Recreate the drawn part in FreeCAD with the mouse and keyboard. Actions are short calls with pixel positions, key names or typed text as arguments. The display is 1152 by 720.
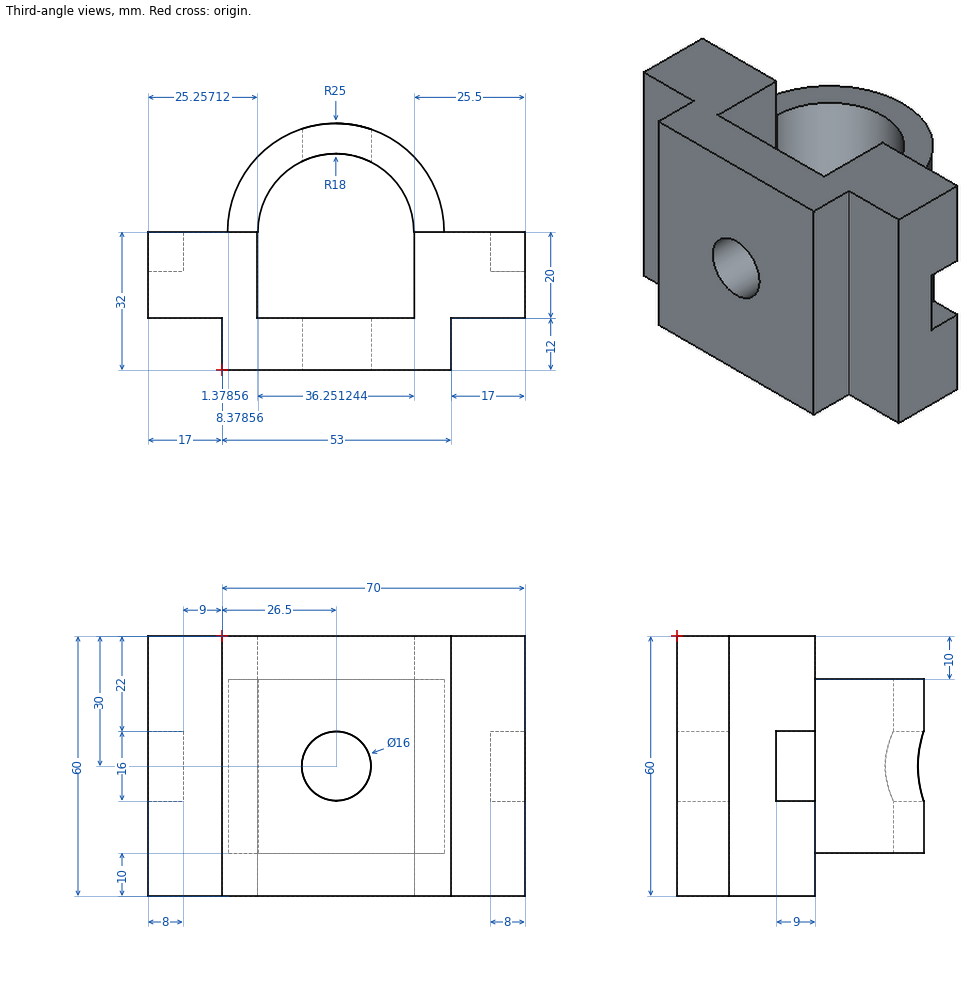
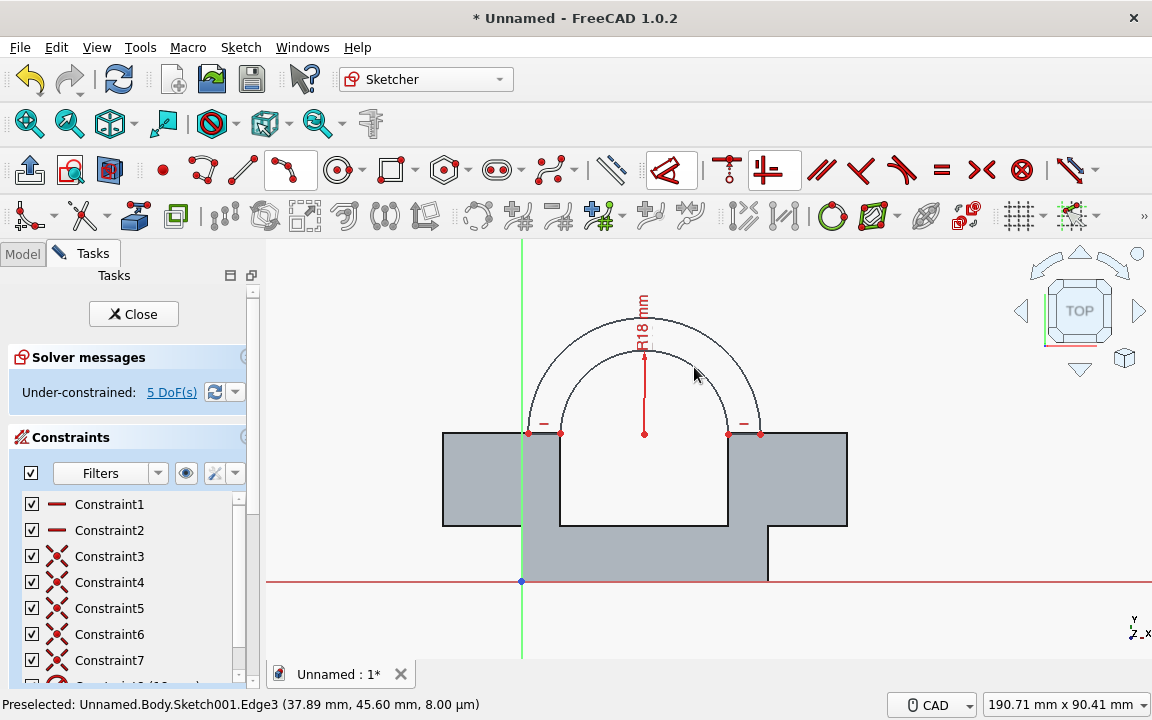
click(713, 340)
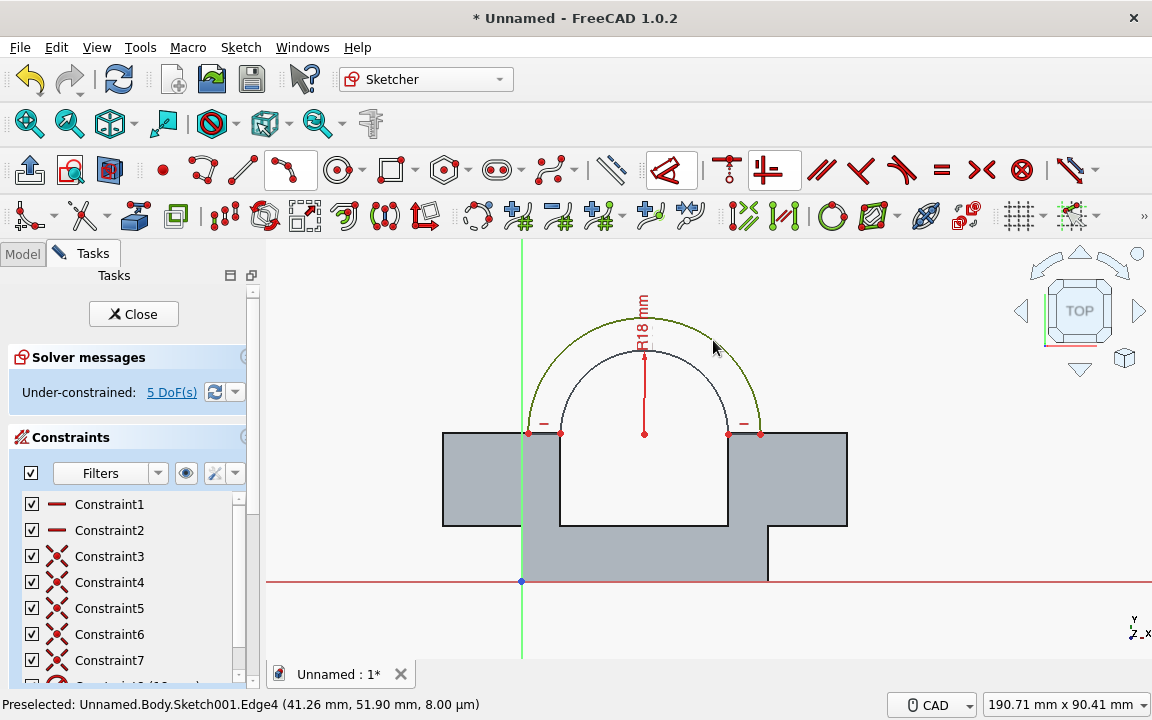
key(k)
key(r)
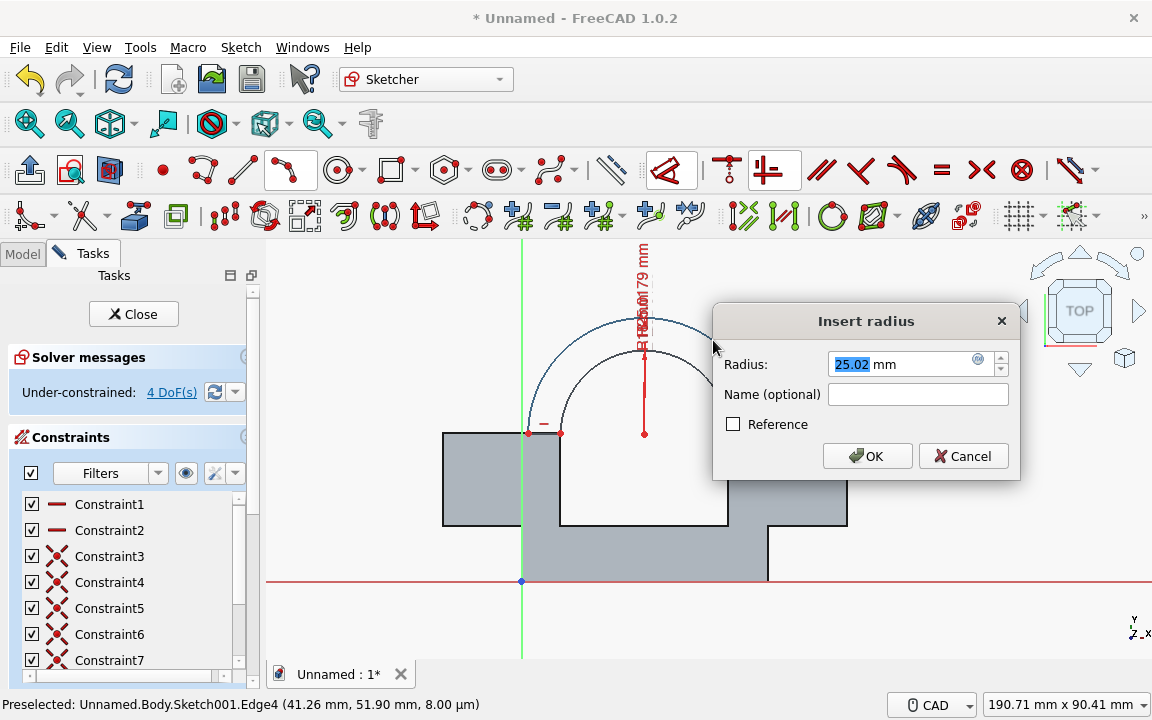
text(25)
key(Return)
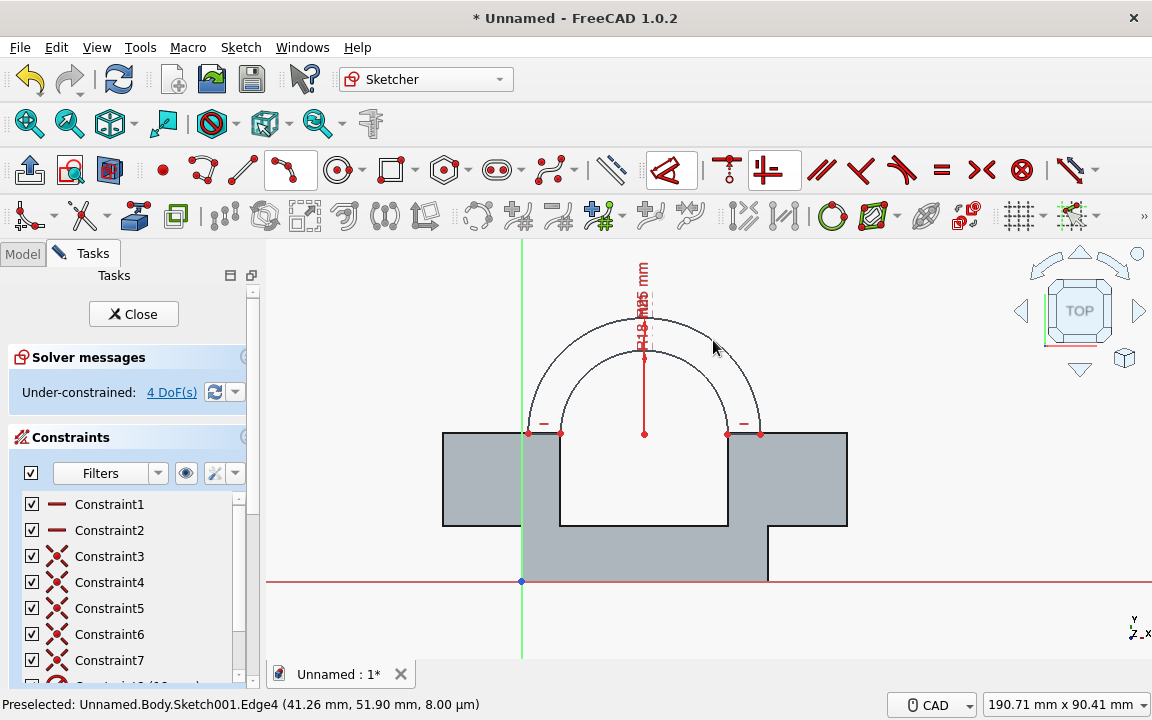
click(528, 434)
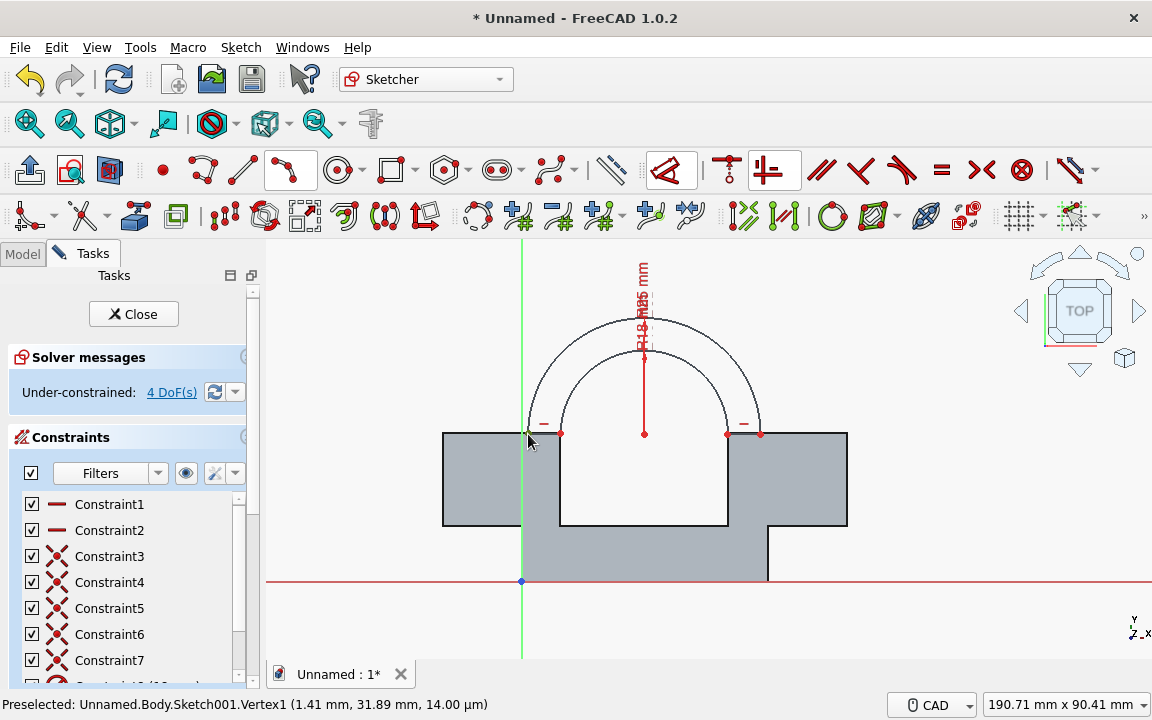
key(i)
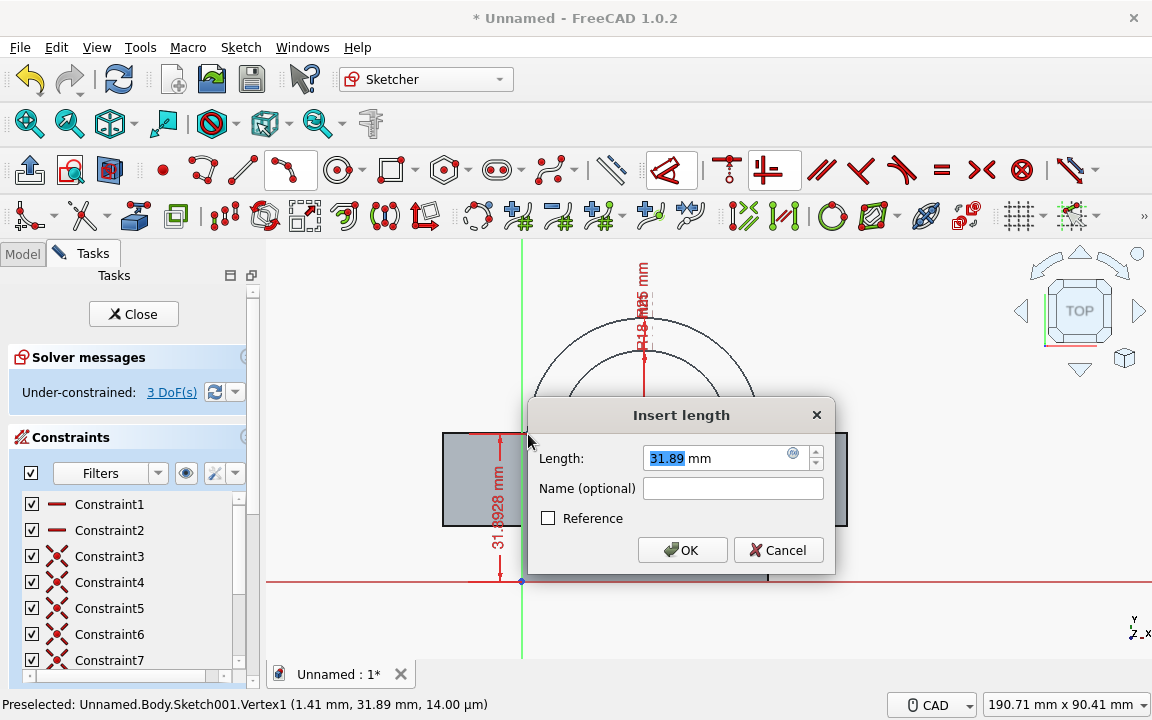
text(32)
key(Return)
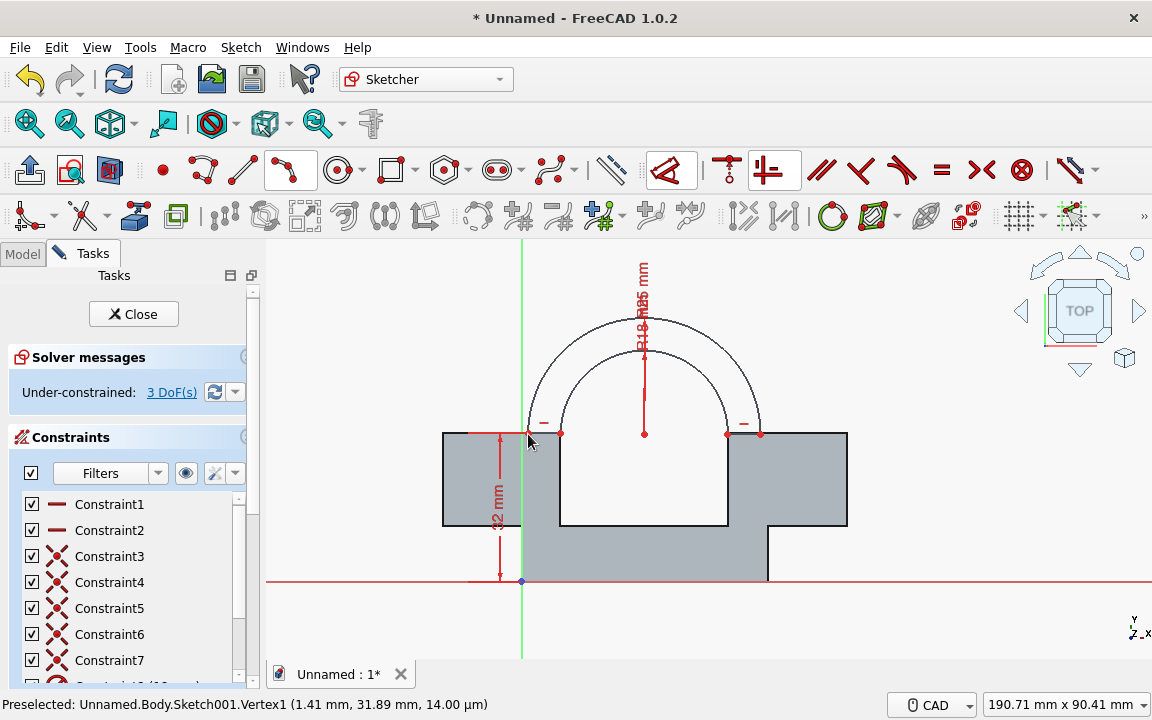
click(728, 434)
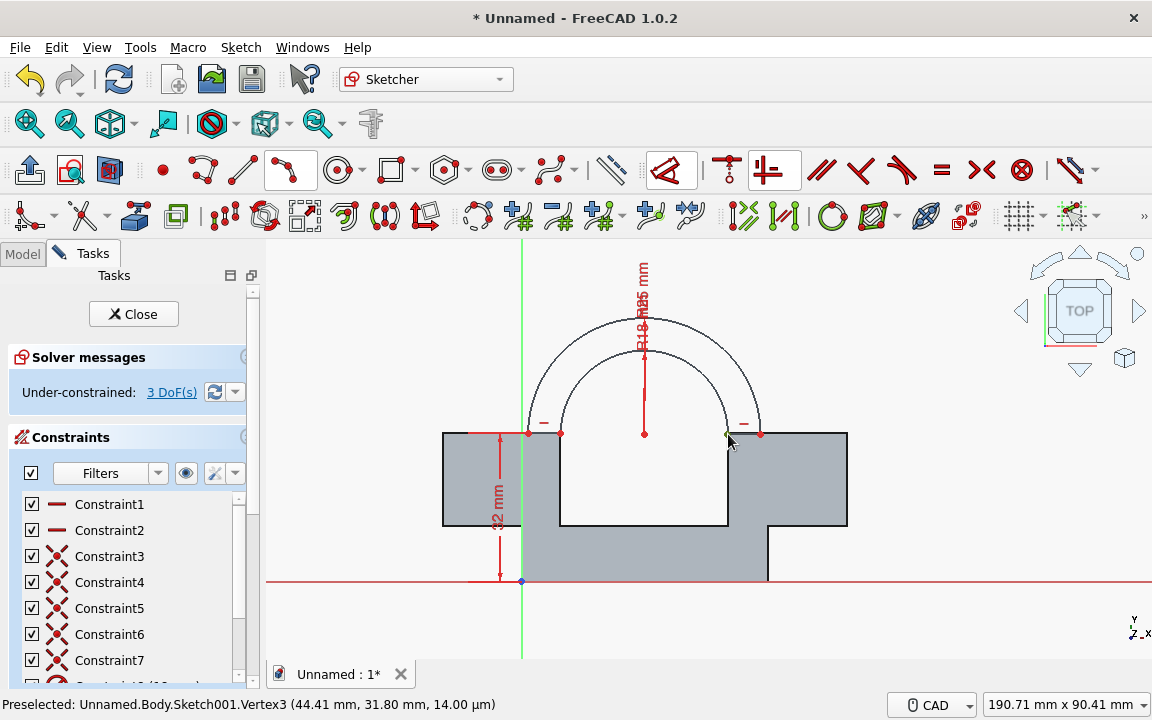
click(692, 170)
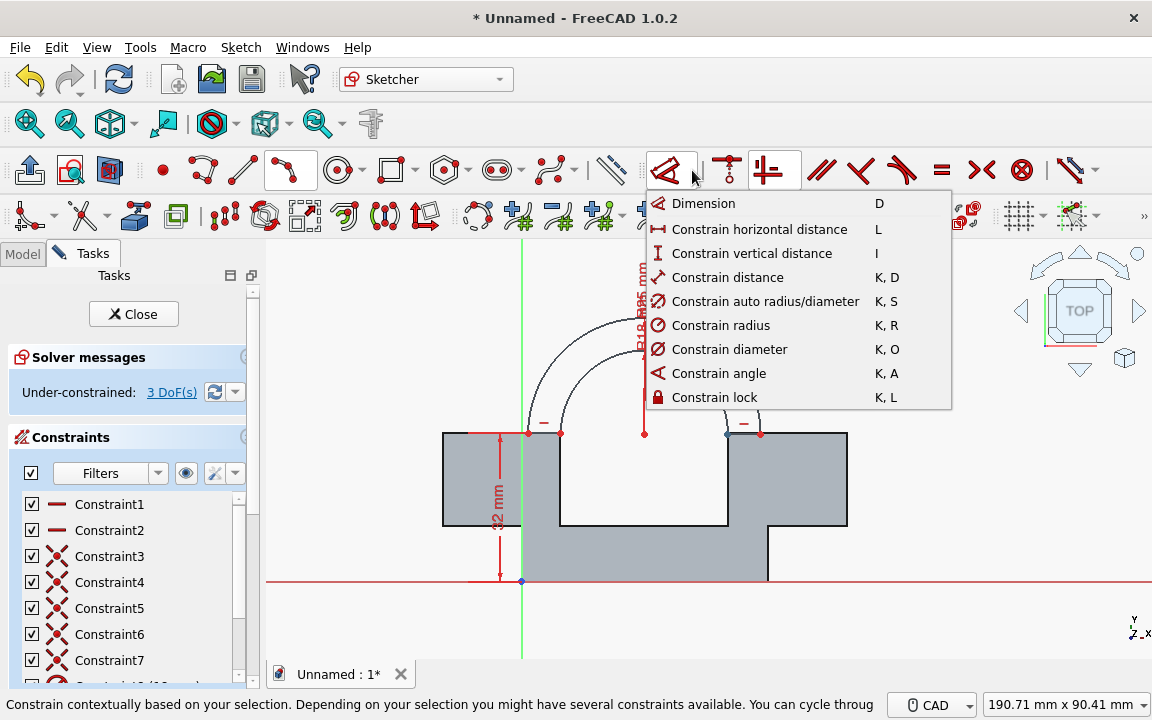
click(799, 253)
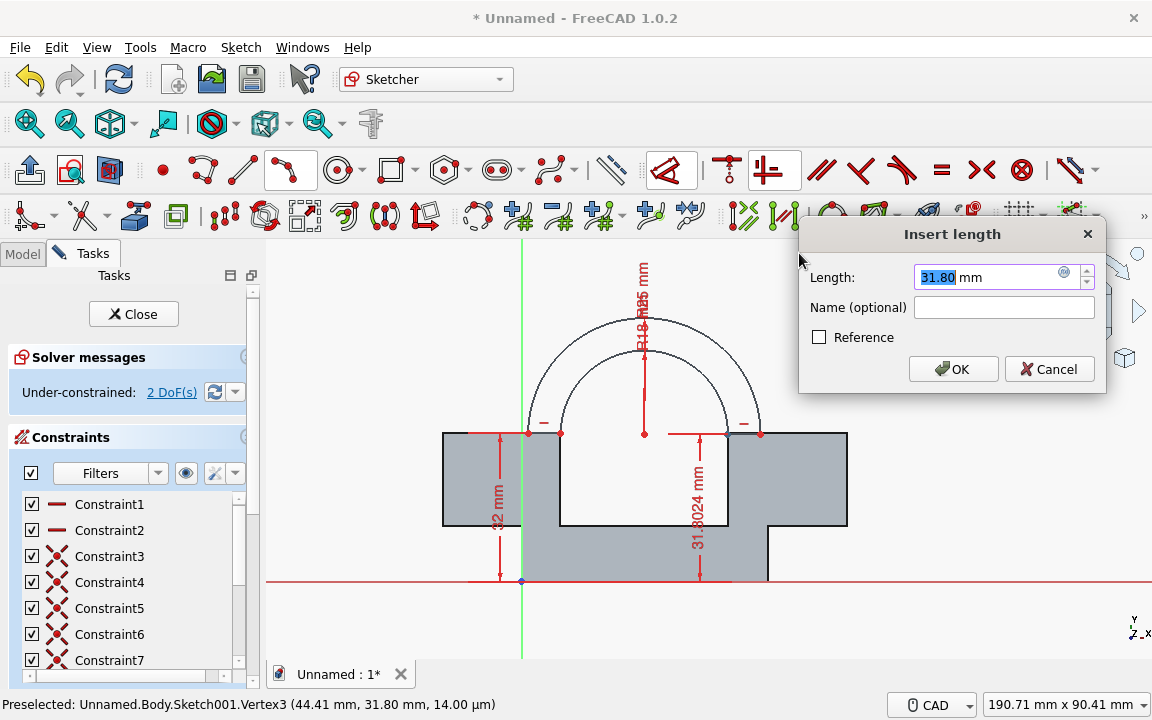
text(32)
key(Return)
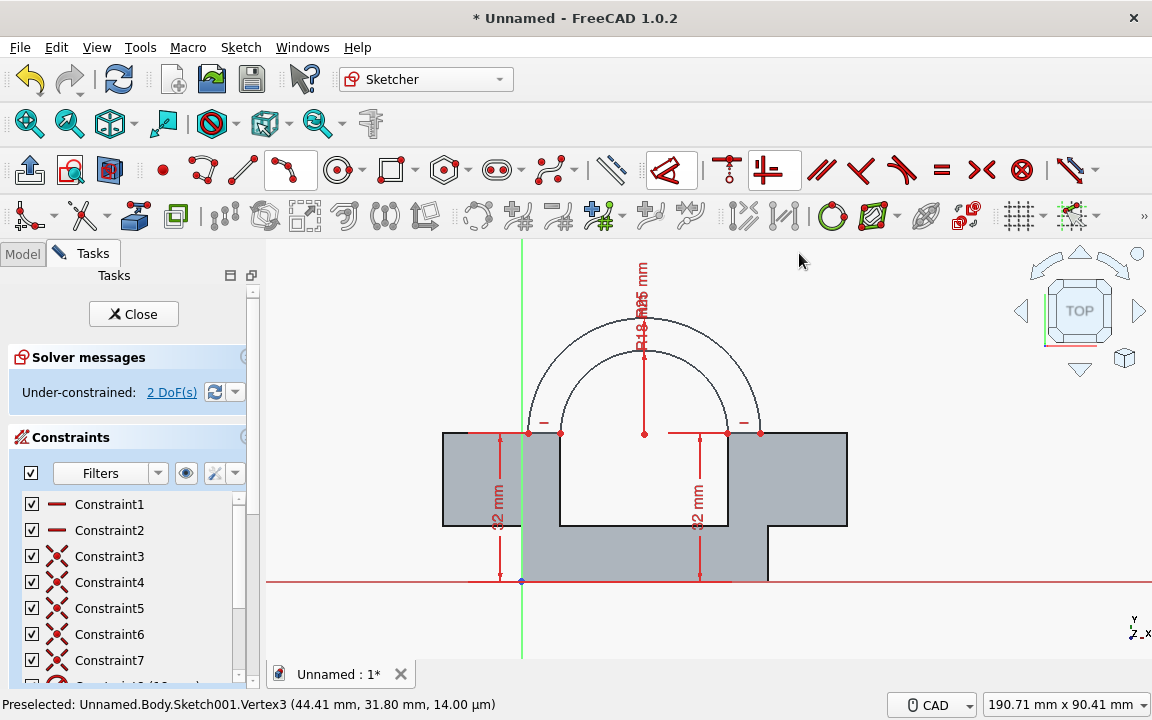
click(644, 434)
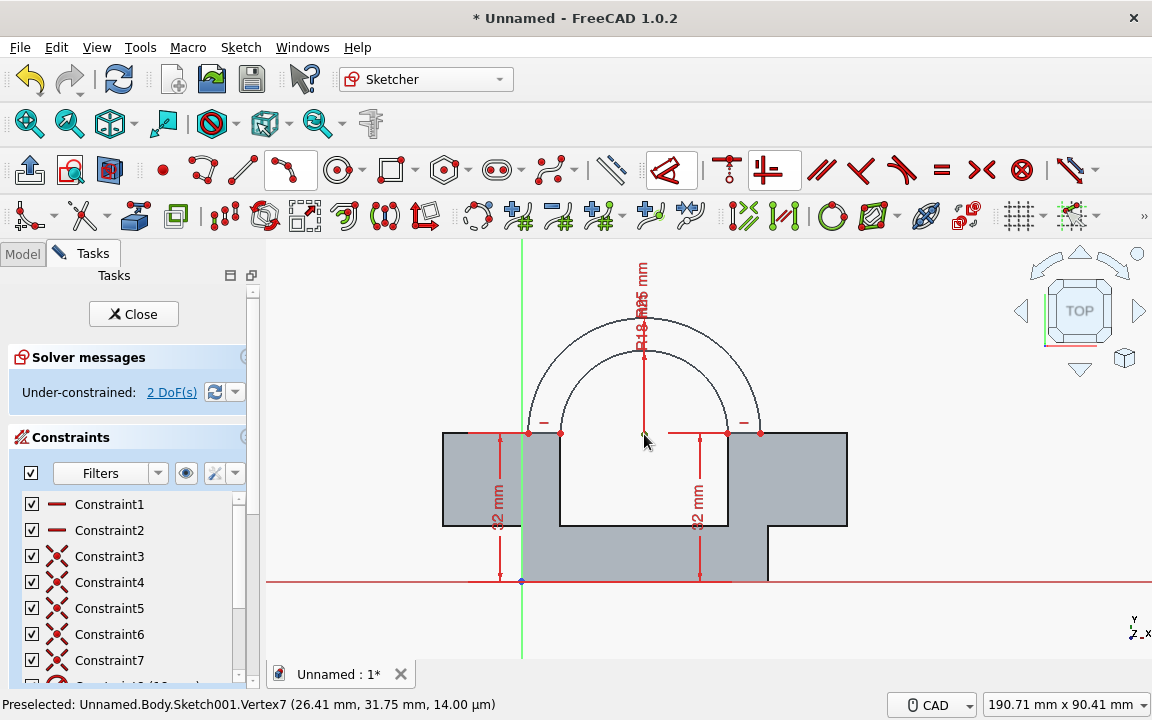
click(692, 170)